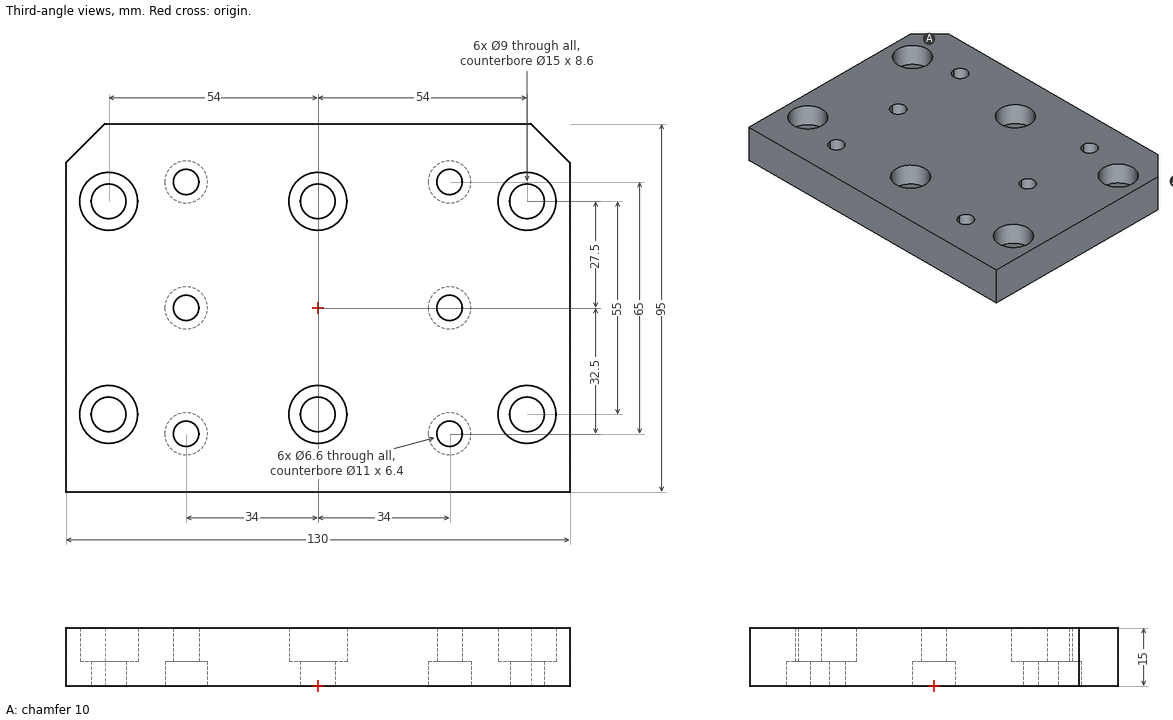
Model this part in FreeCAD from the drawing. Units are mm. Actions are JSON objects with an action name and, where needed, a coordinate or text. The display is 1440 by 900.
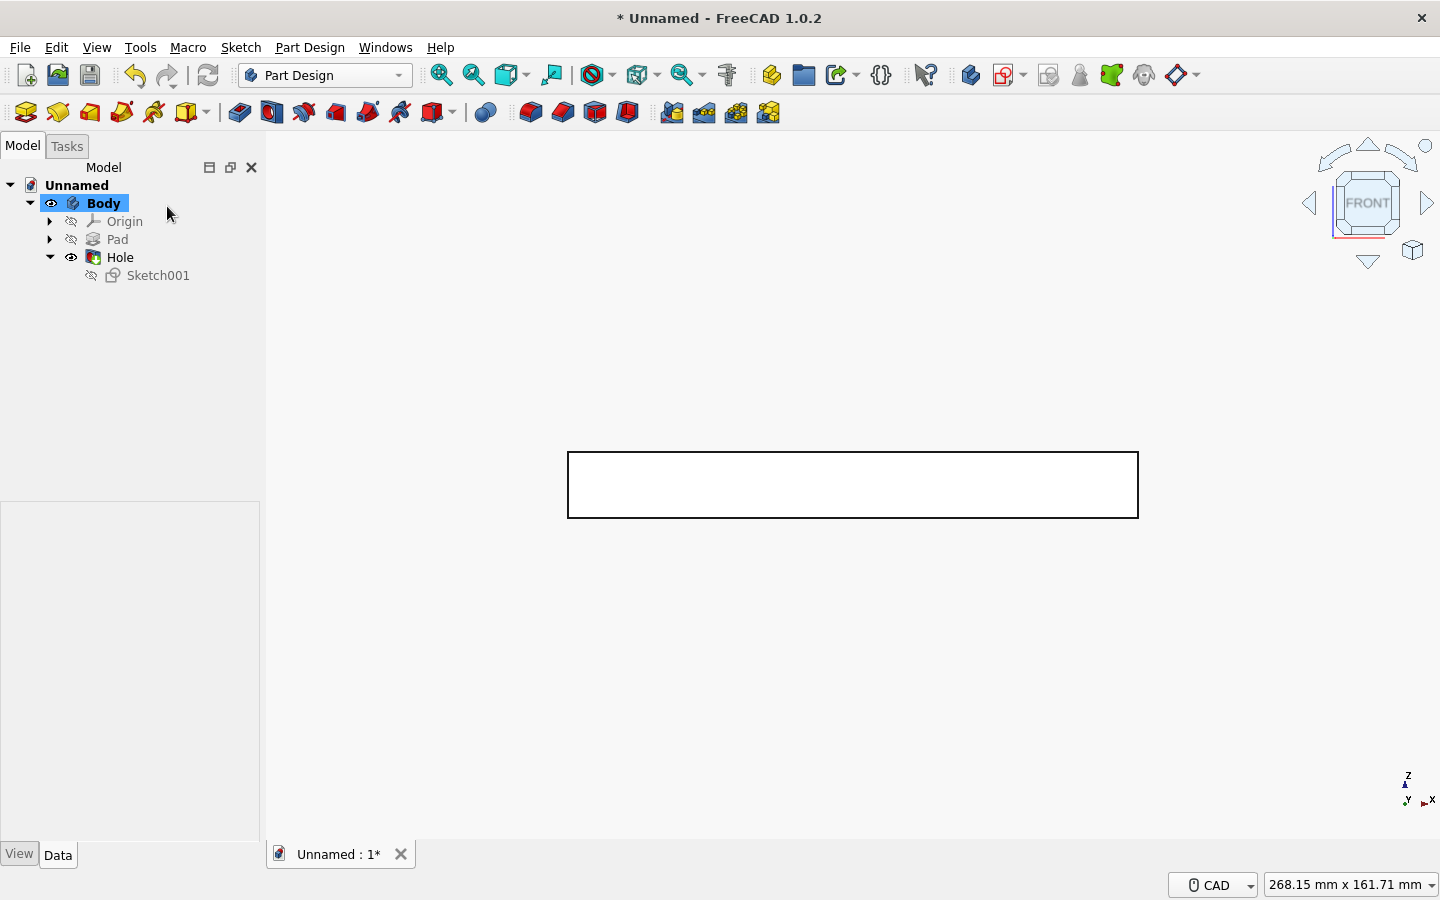
{"action": "key", "text": "3"}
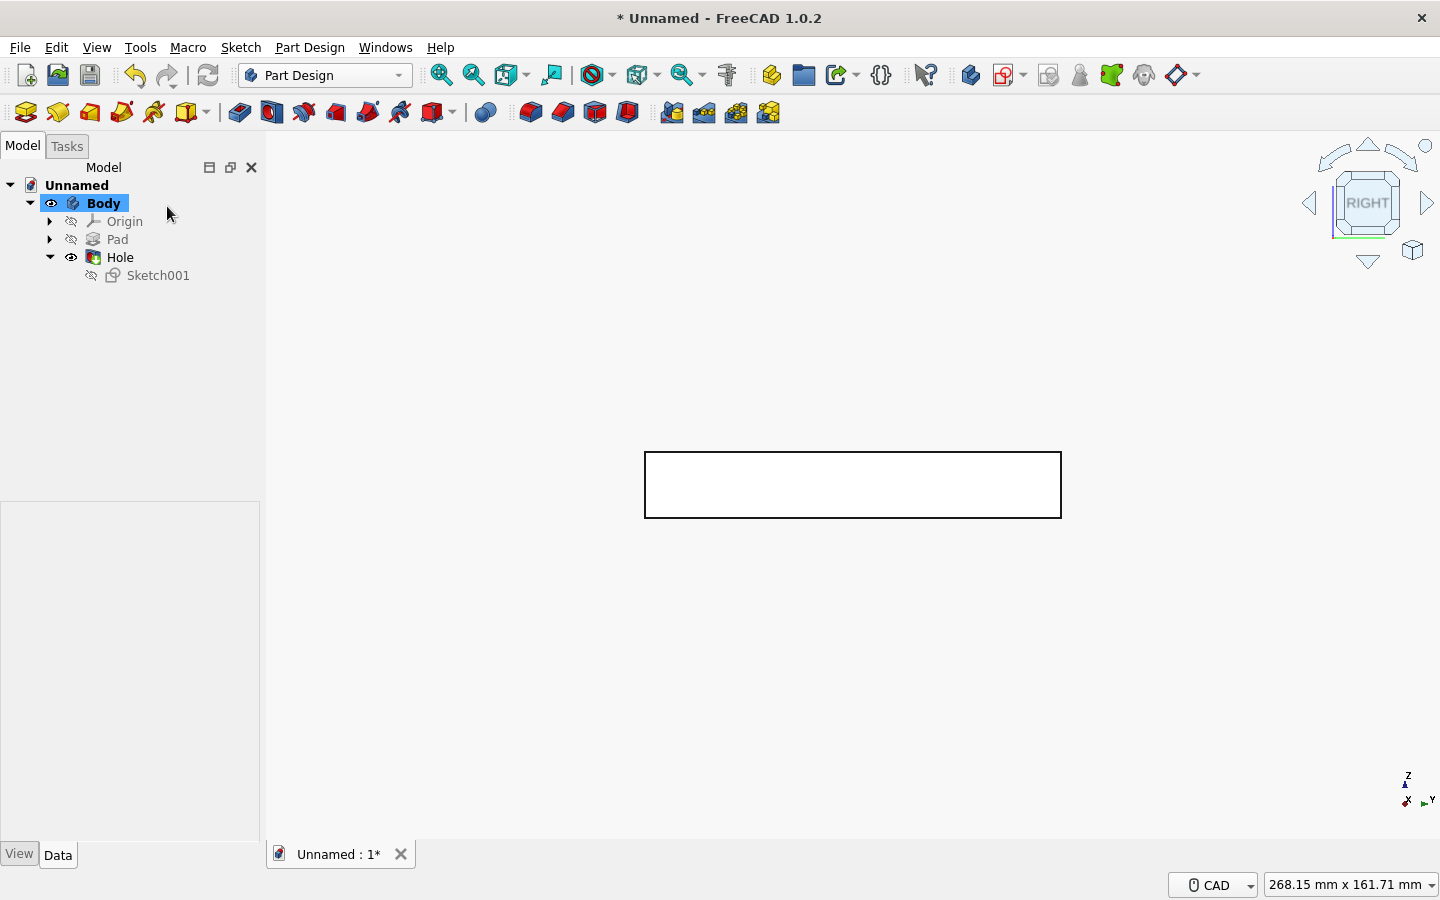
{"action": "left_click", "coordinate": [442, 76]}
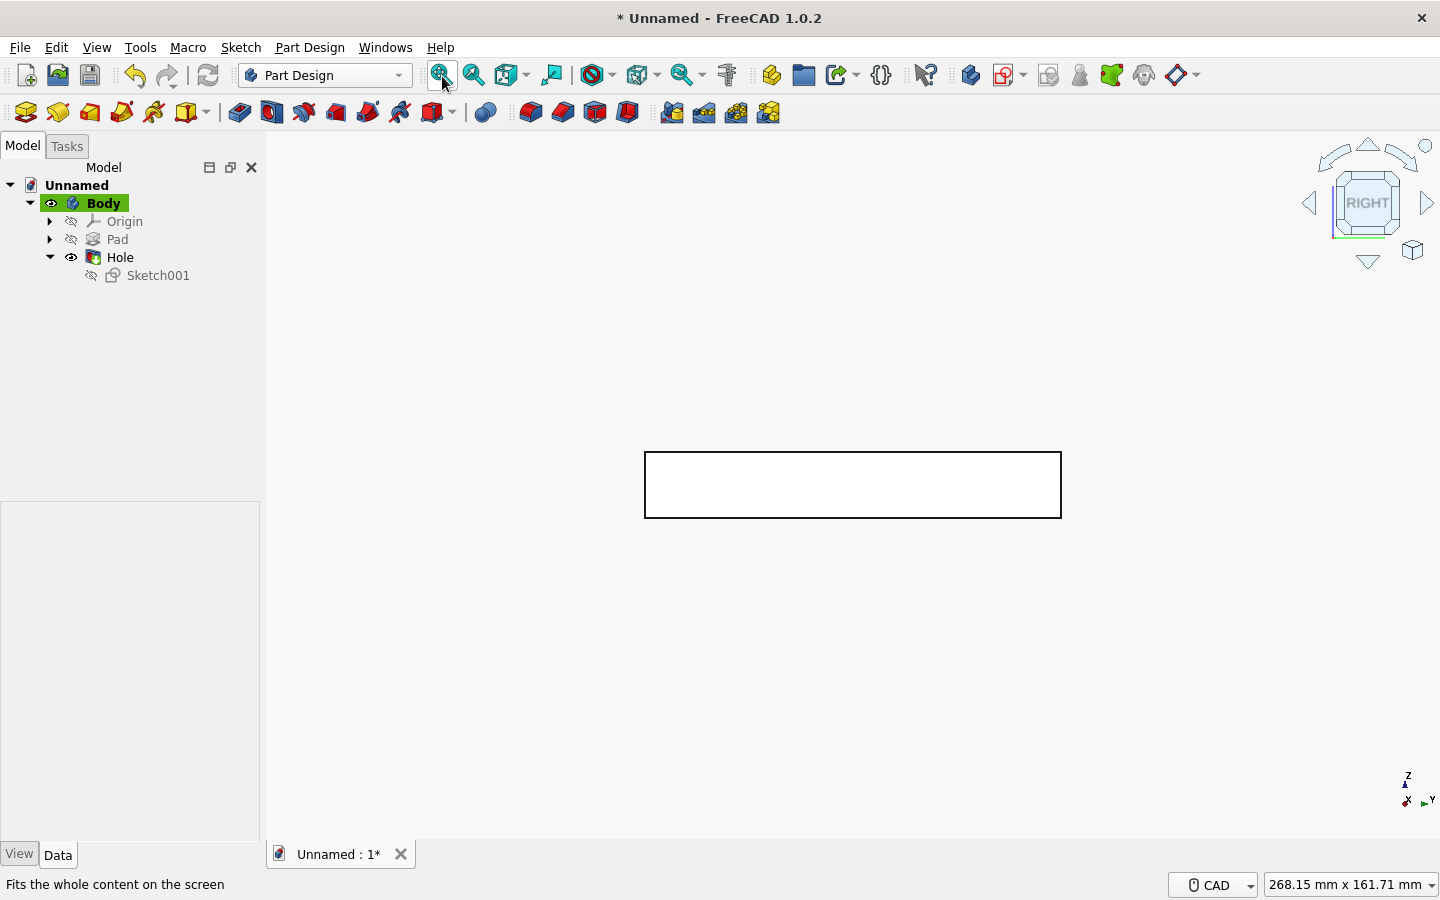
{"action": "left_click", "coordinate": [1061, 484]}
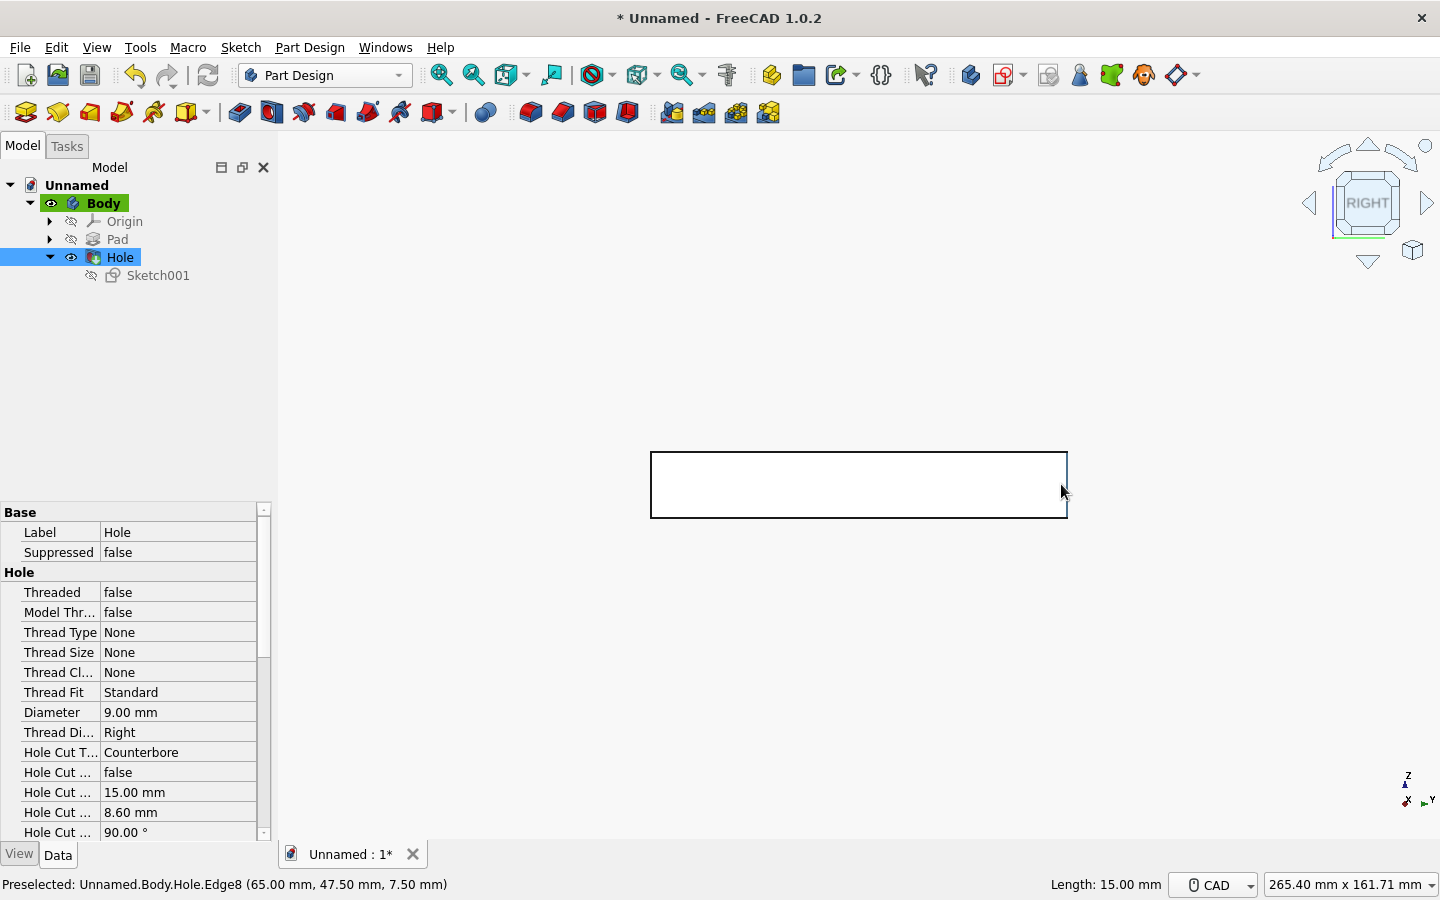
{"action": "key", "text": "5"}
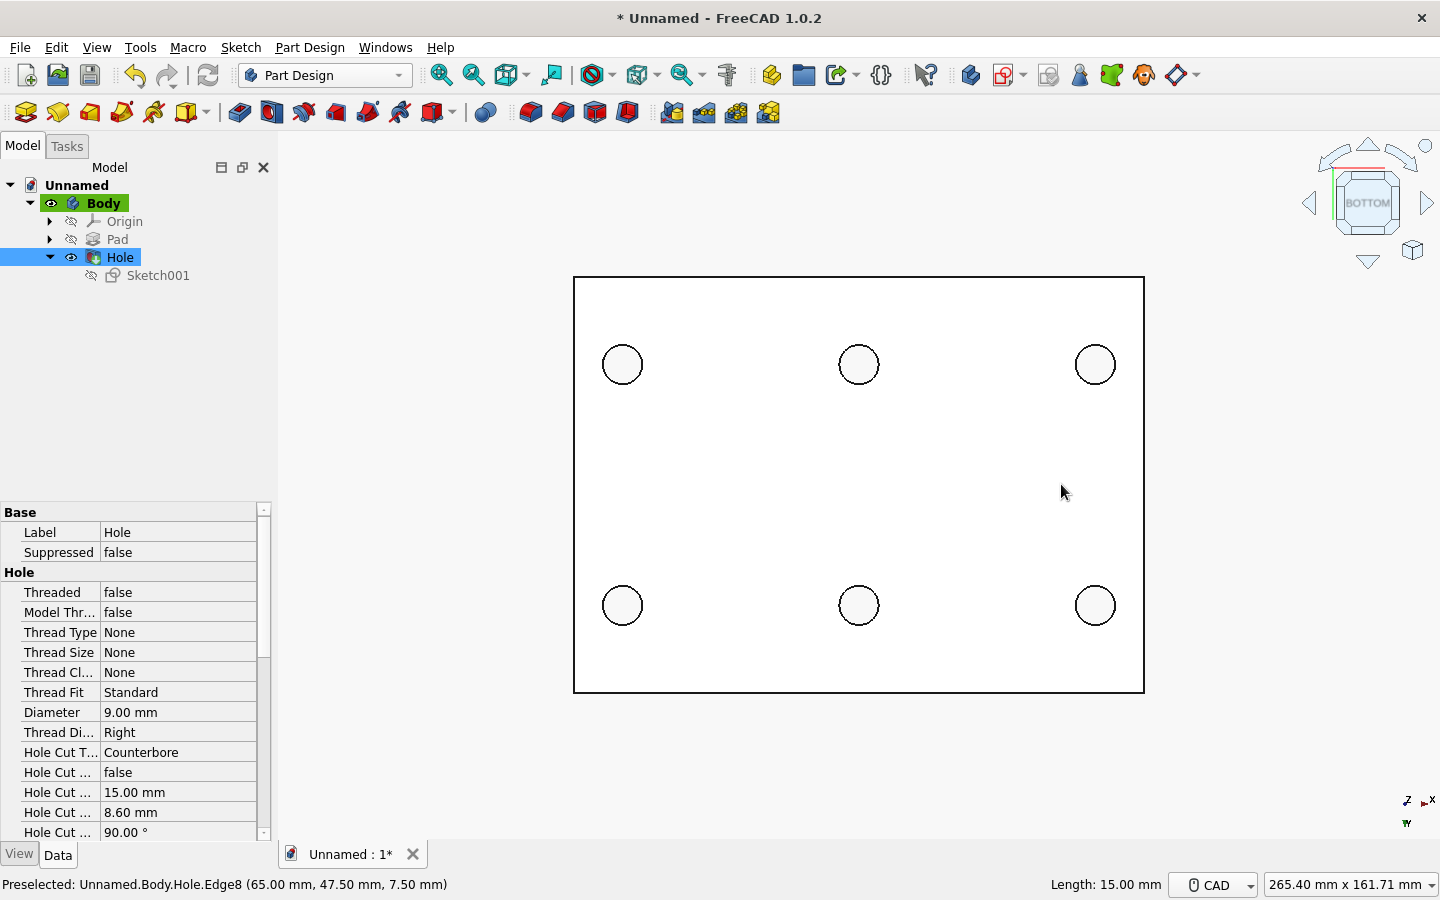
{"action": "key", "text": "4"}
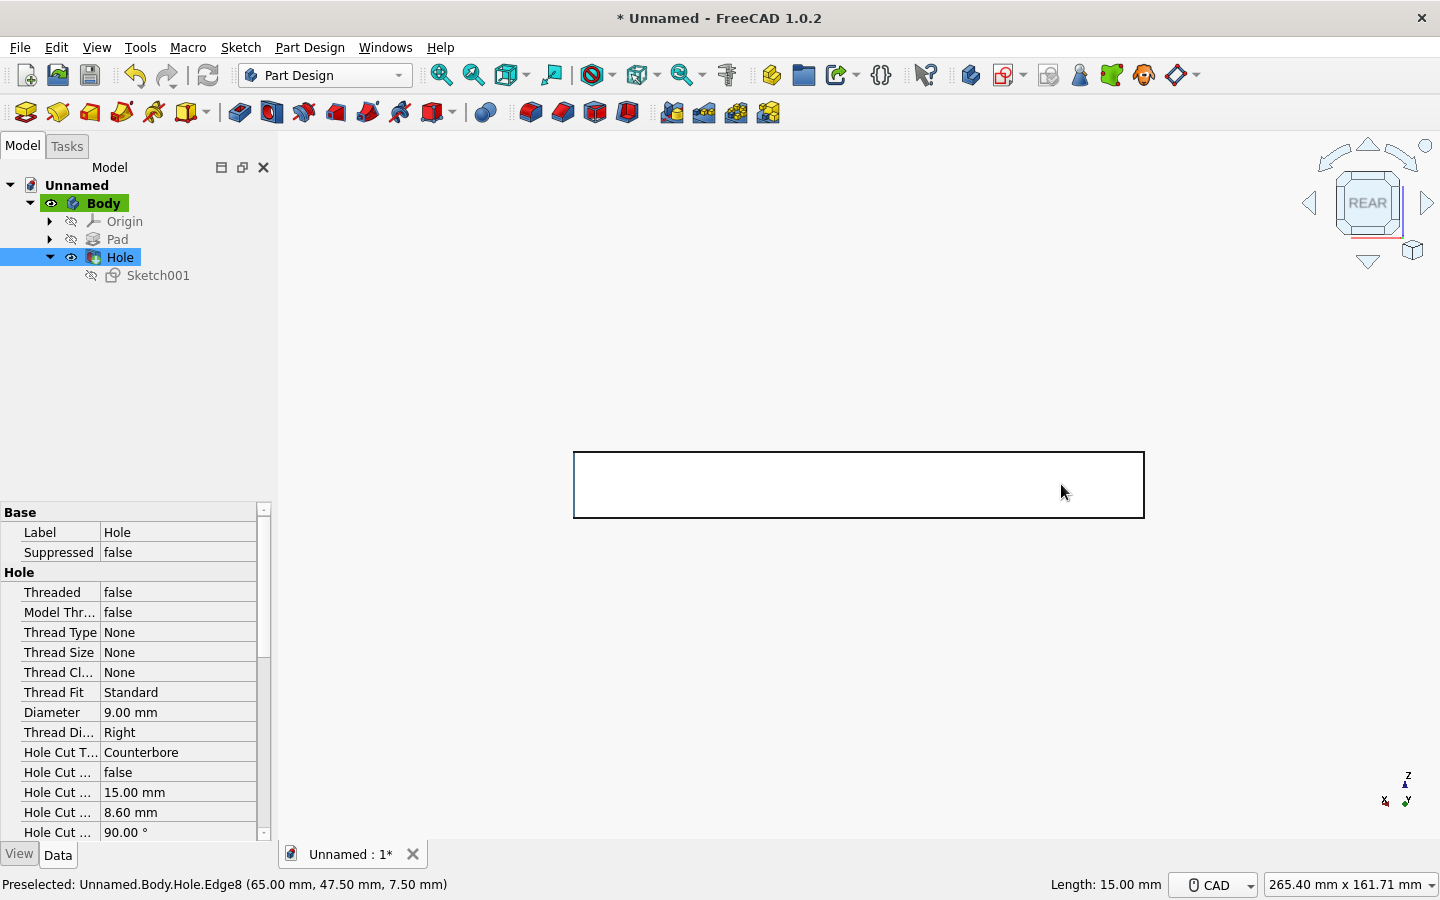
{"action": "left_click", "coordinate": [1144, 484], "text": "ctrl"}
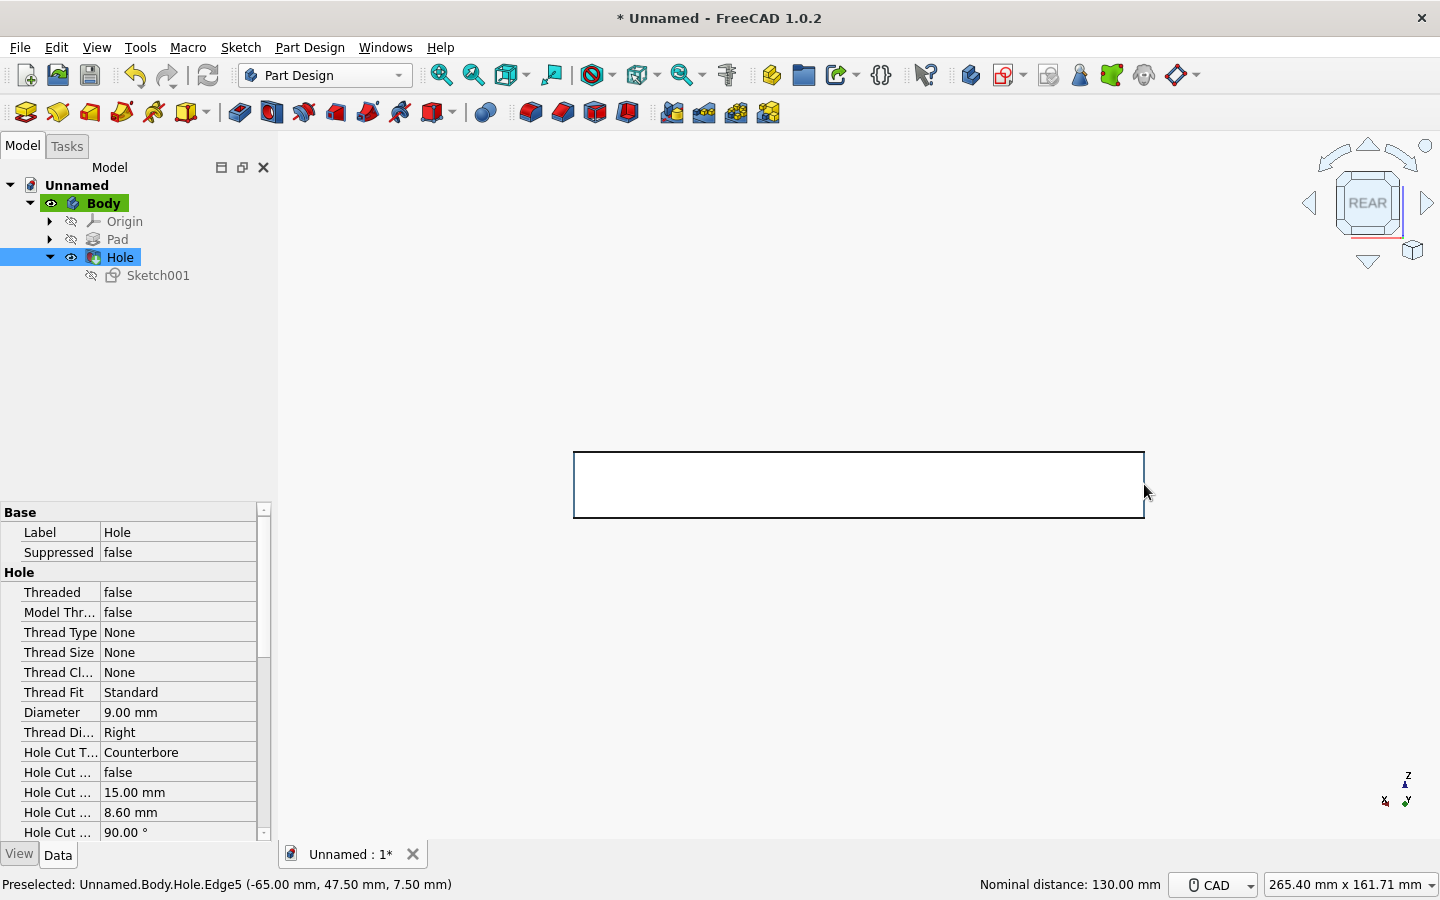
{"action": "left_click", "coordinate": [564, 112]}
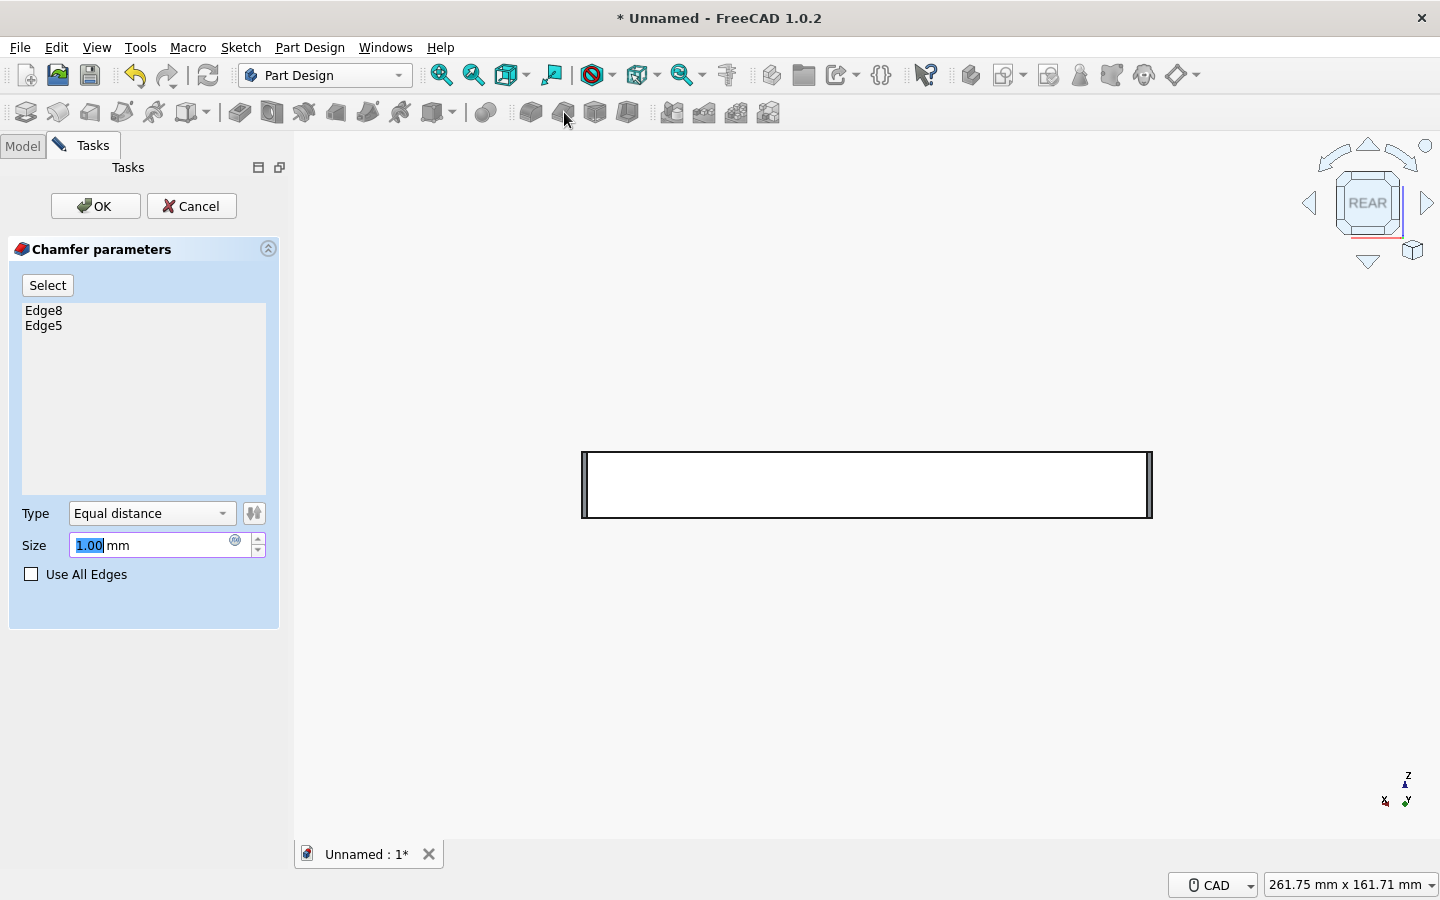
{"action": "type", "text": "10"}
{"action": "key", "text": "Tab"}